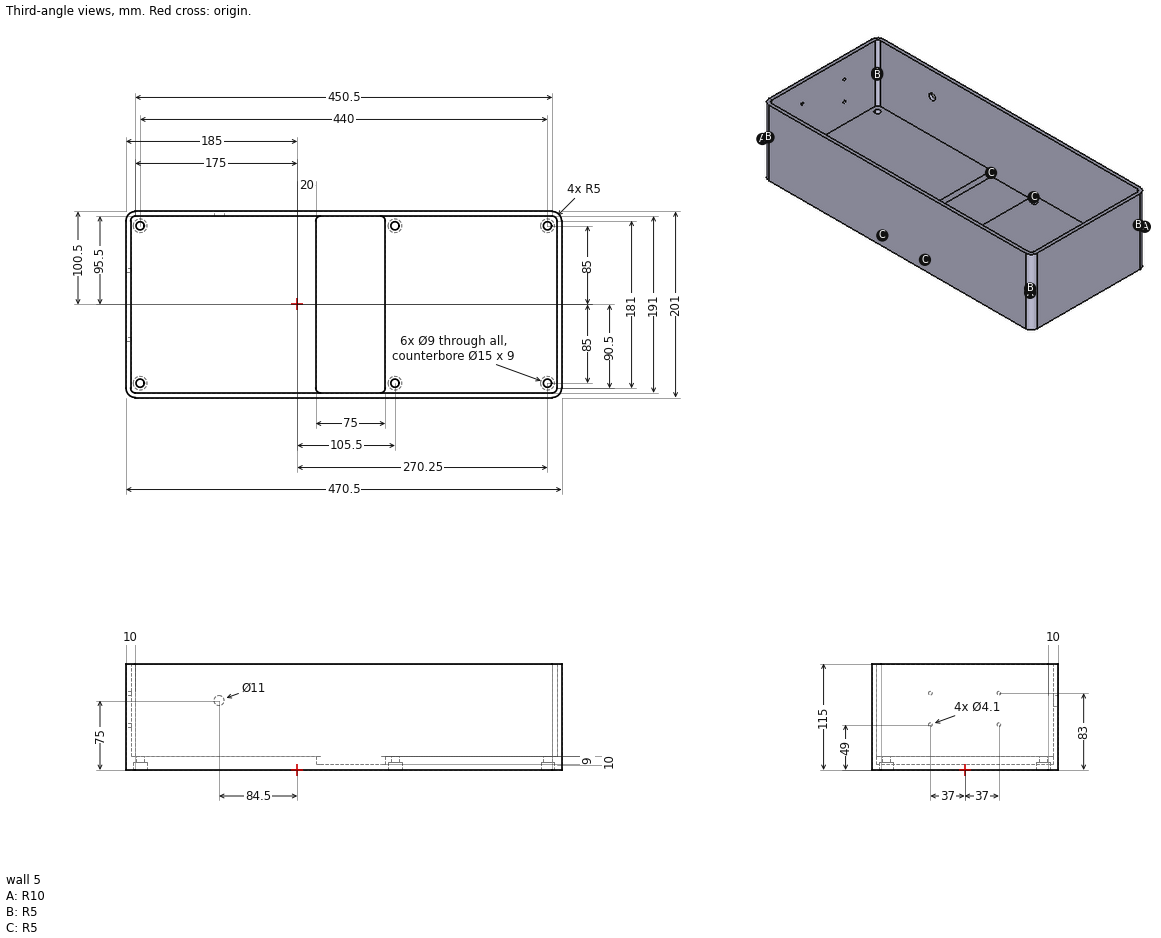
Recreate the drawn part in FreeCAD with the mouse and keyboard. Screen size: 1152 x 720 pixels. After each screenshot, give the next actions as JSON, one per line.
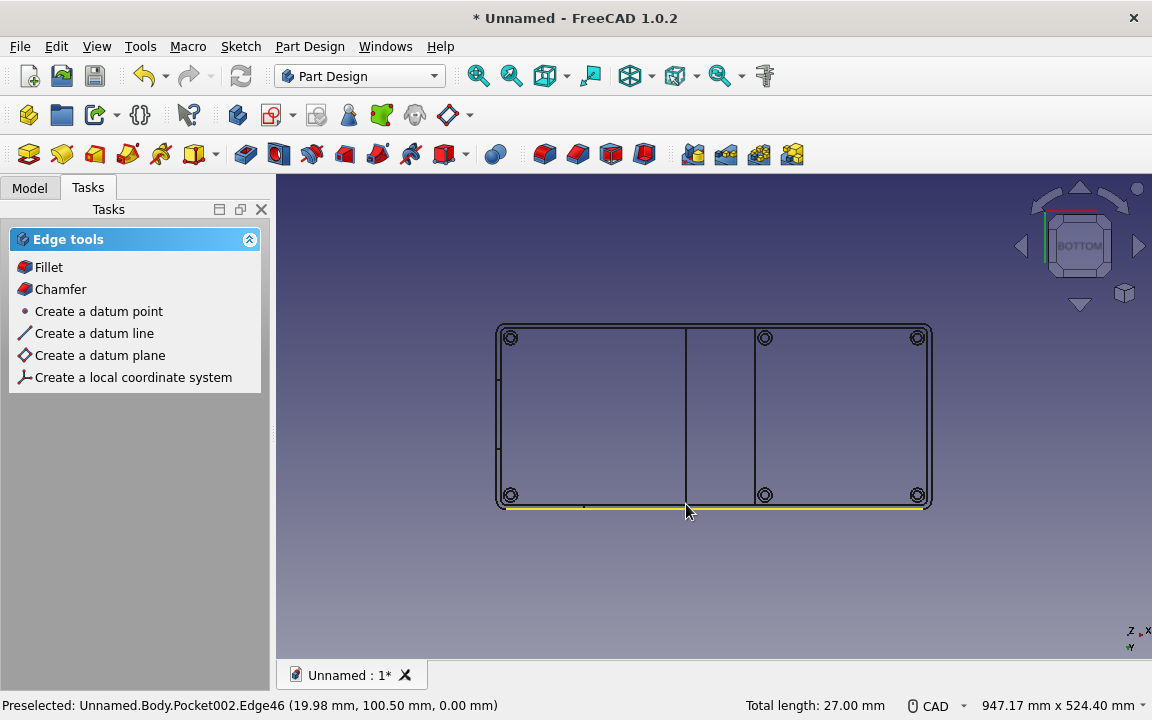
{"action": "key", "text": "4"}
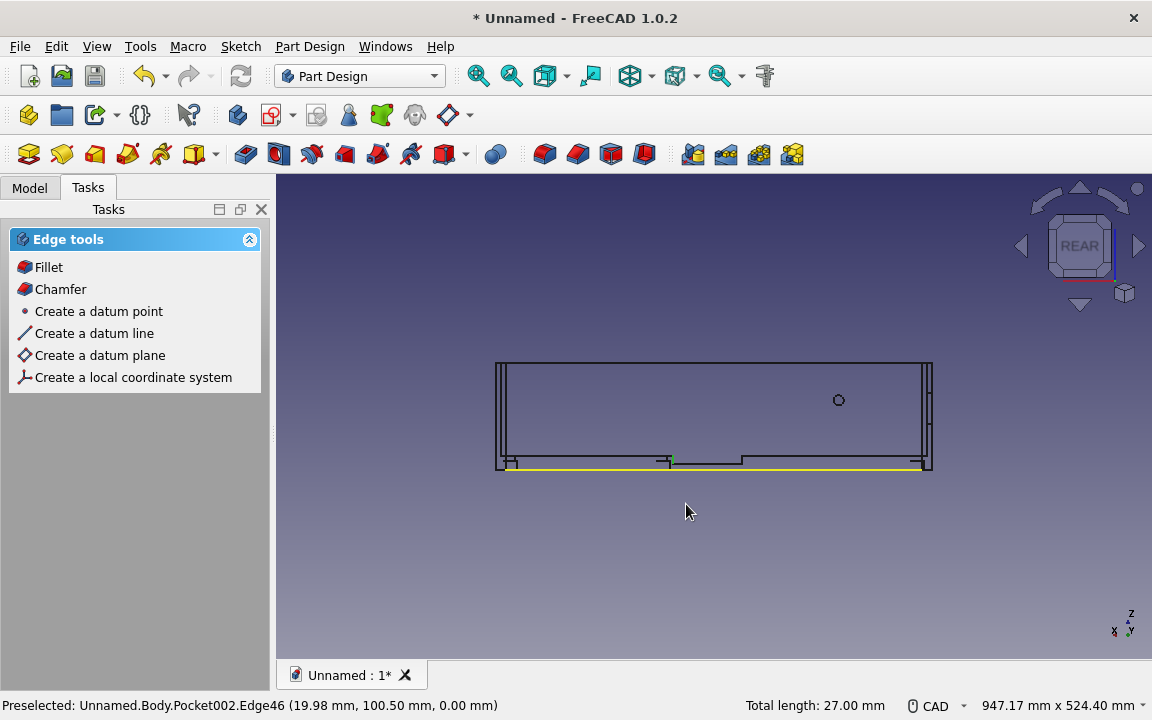
{"action": "left_click", "coordinate": [742, 461], "text": "ctrl"}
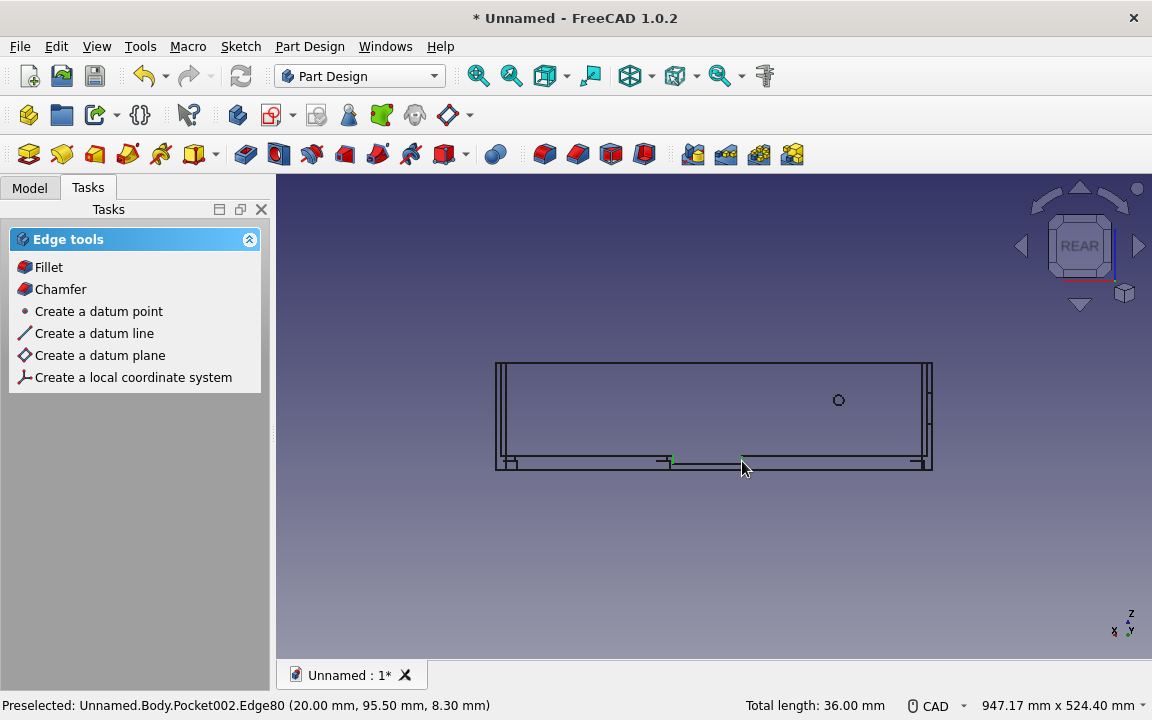
{"action": "key", "text": "v 1"}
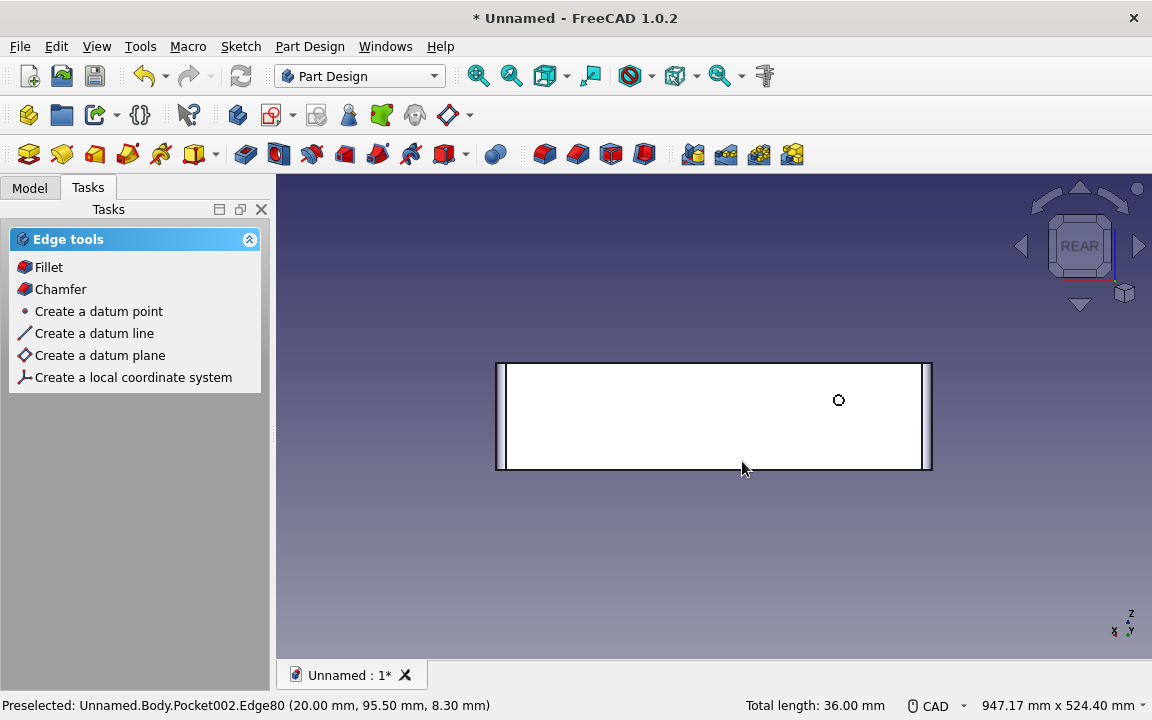
{"action": "left_click", "coordinate": [545, 154]}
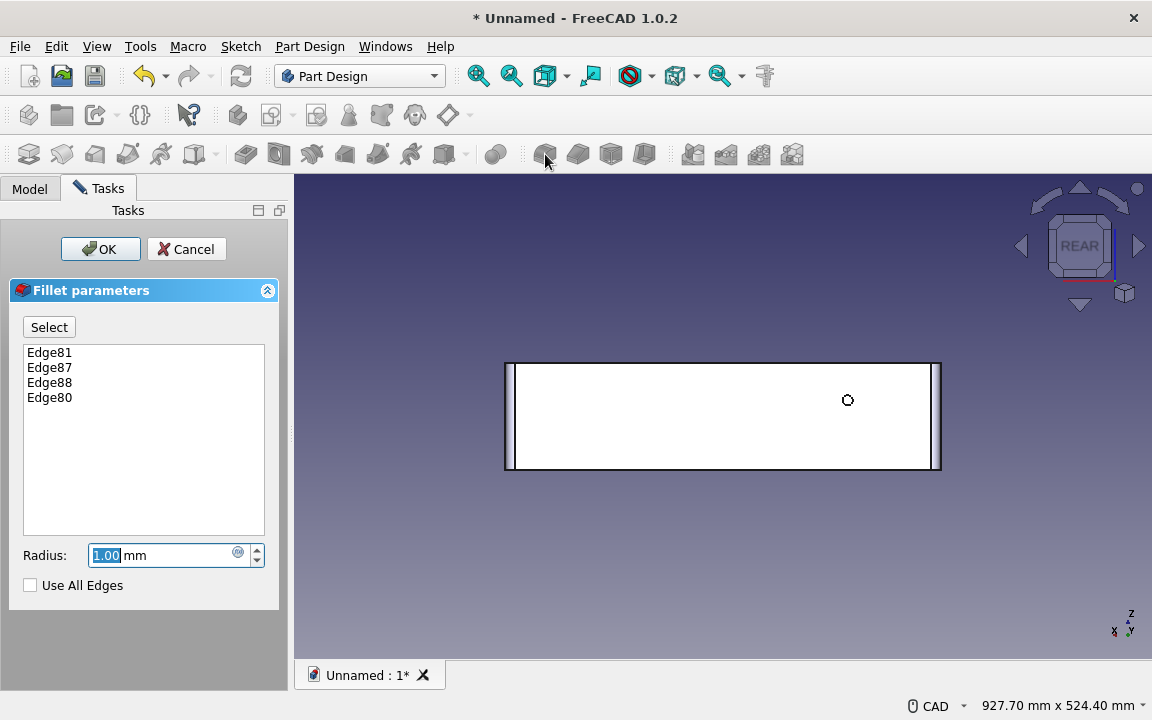
{"action": "type", "text": "5"}
{"action": "key", "text": "Tab"}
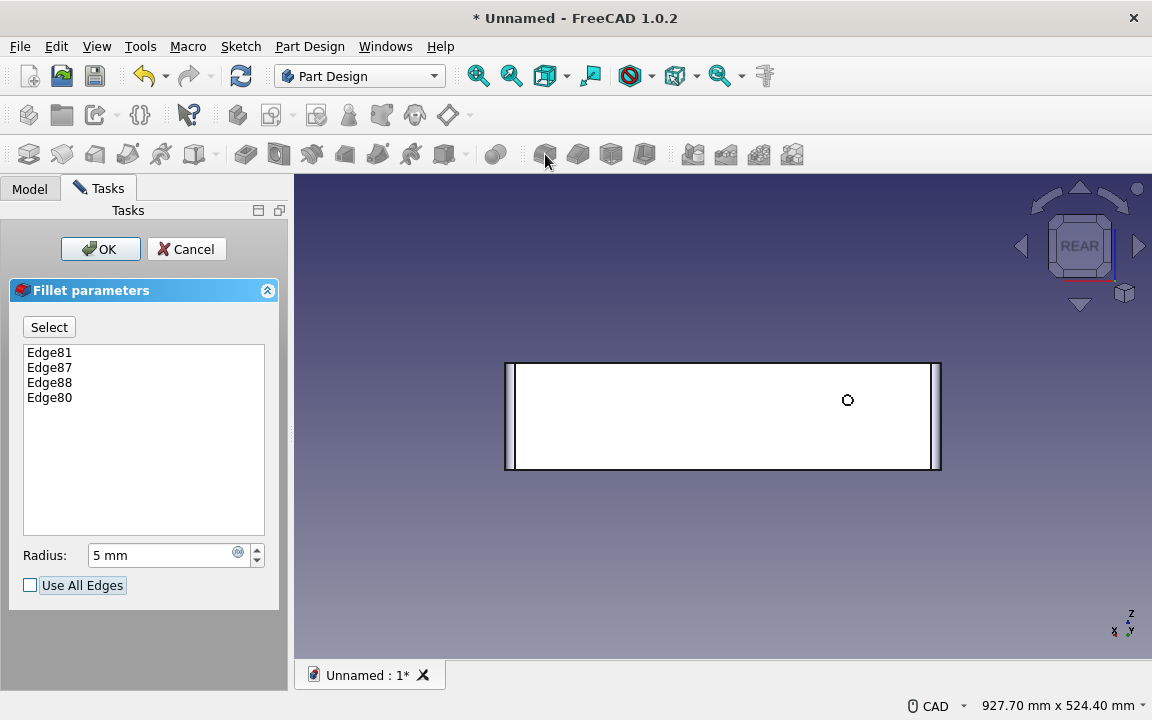
{"action": "left_click", "coordinate": [101, 249]}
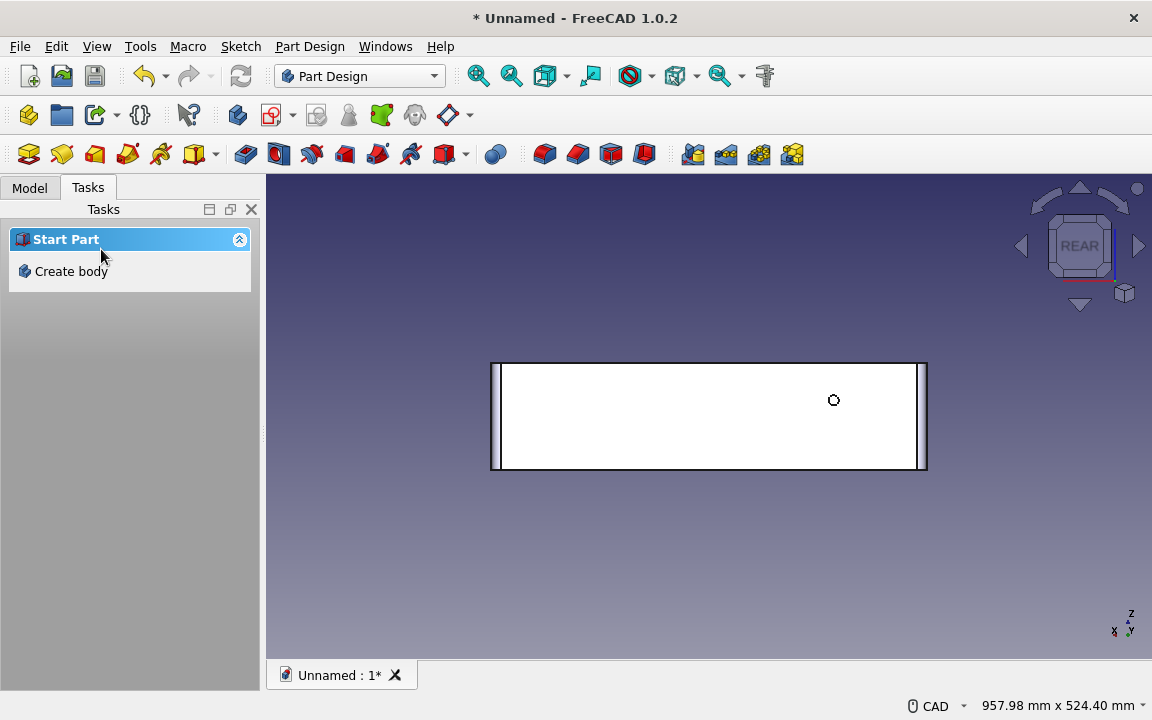
{"action": "key", "text": "0"}